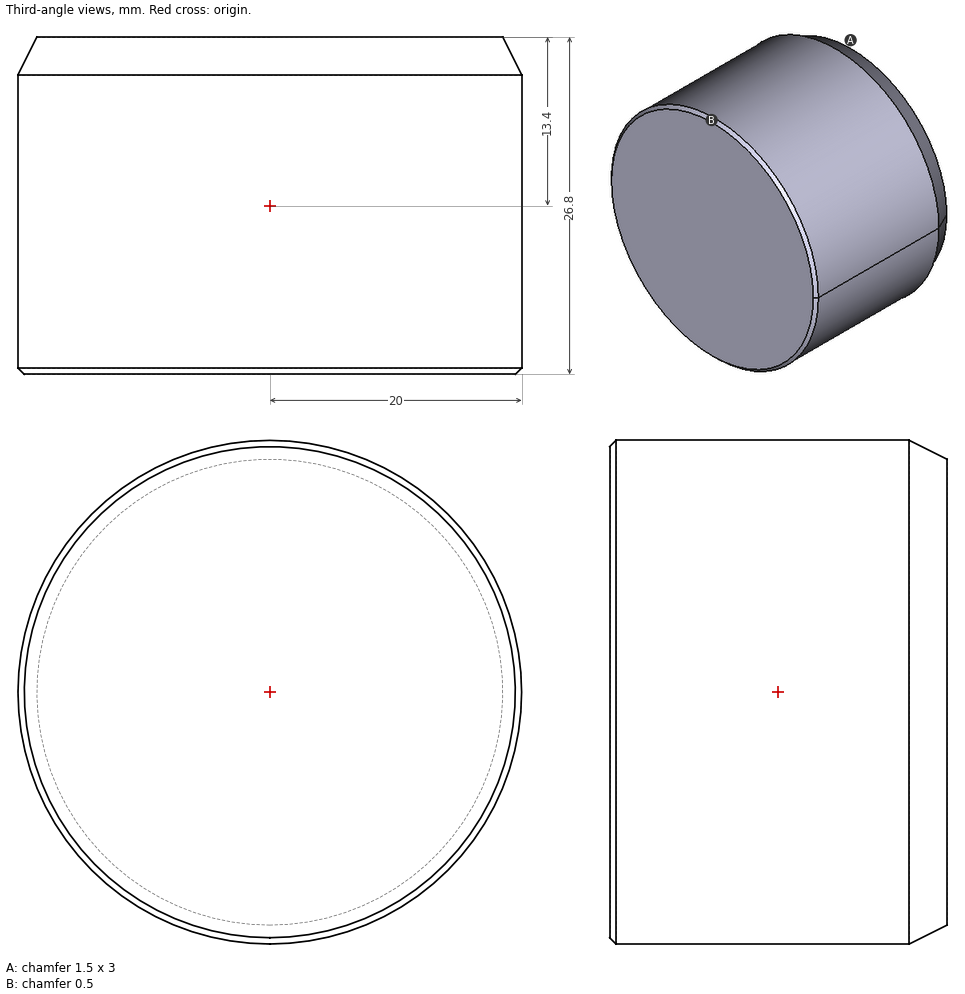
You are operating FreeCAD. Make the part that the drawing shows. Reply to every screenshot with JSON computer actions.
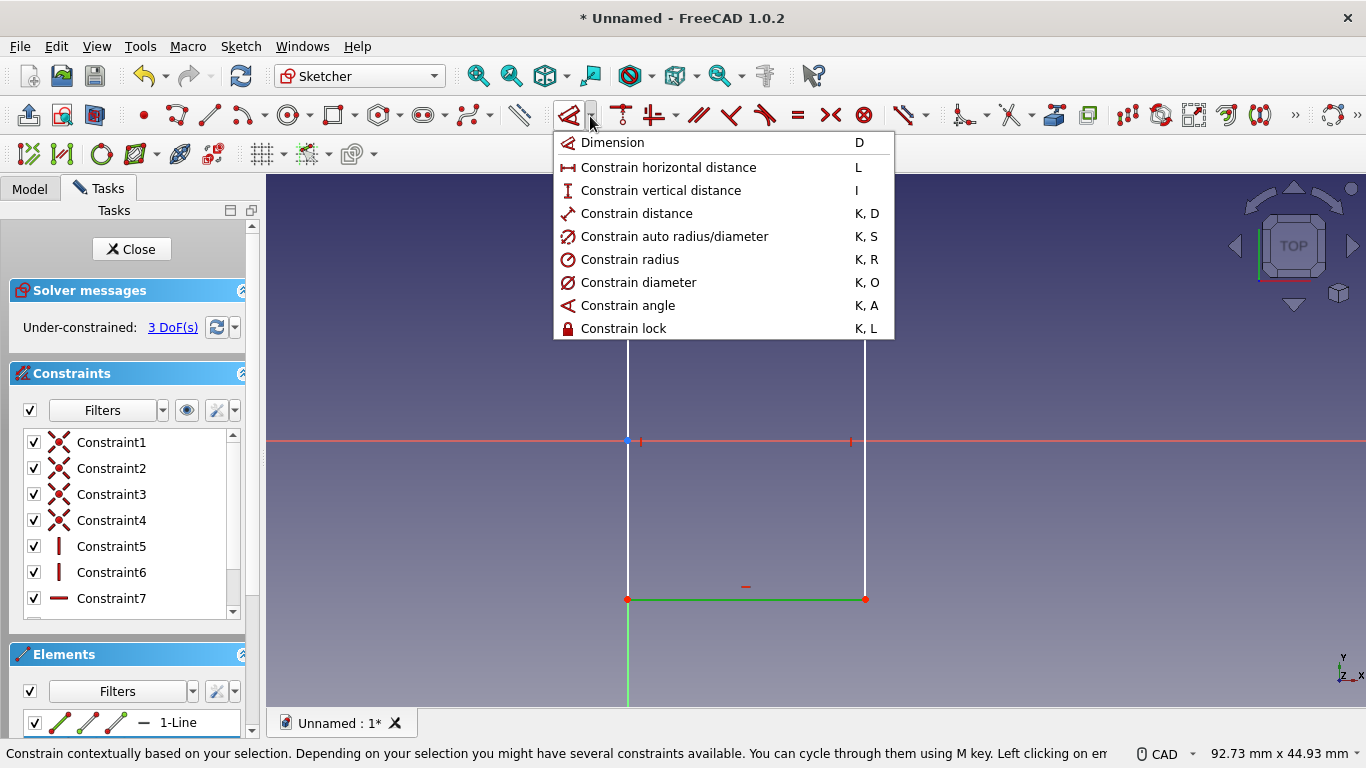
{"action": "left_click", "coordinate": [724, 168]}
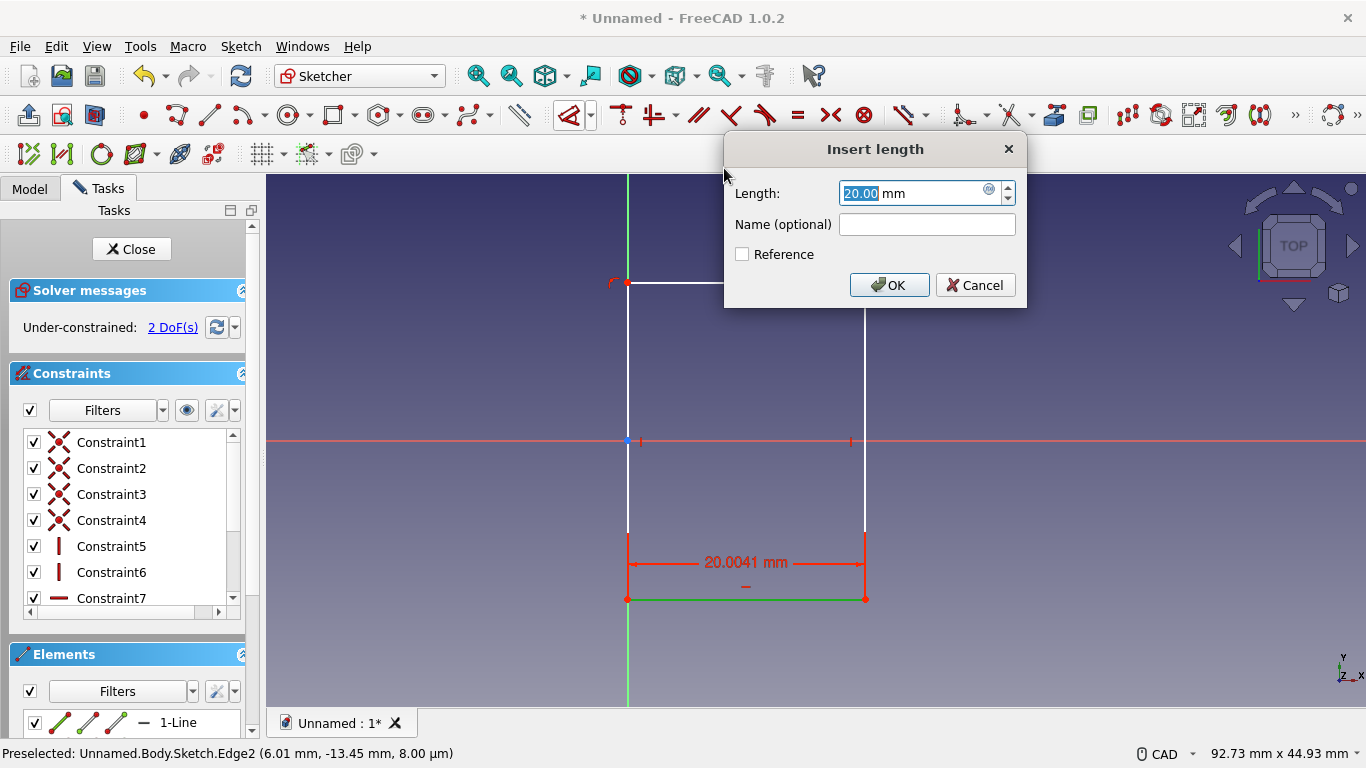
{"action": "type", "text": "20"}
{"action": "key", "text": "Return"}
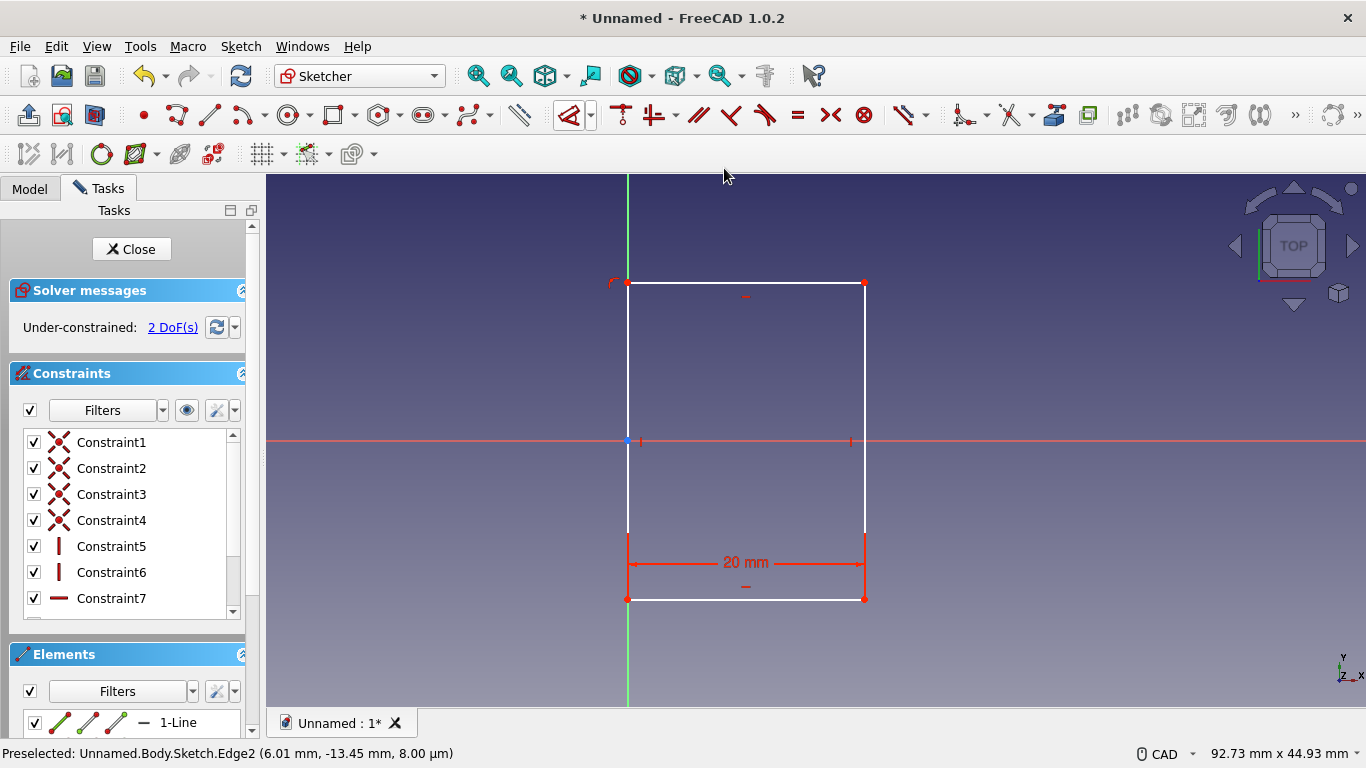
{"action": "left_click", "coordinate": [628, 378]}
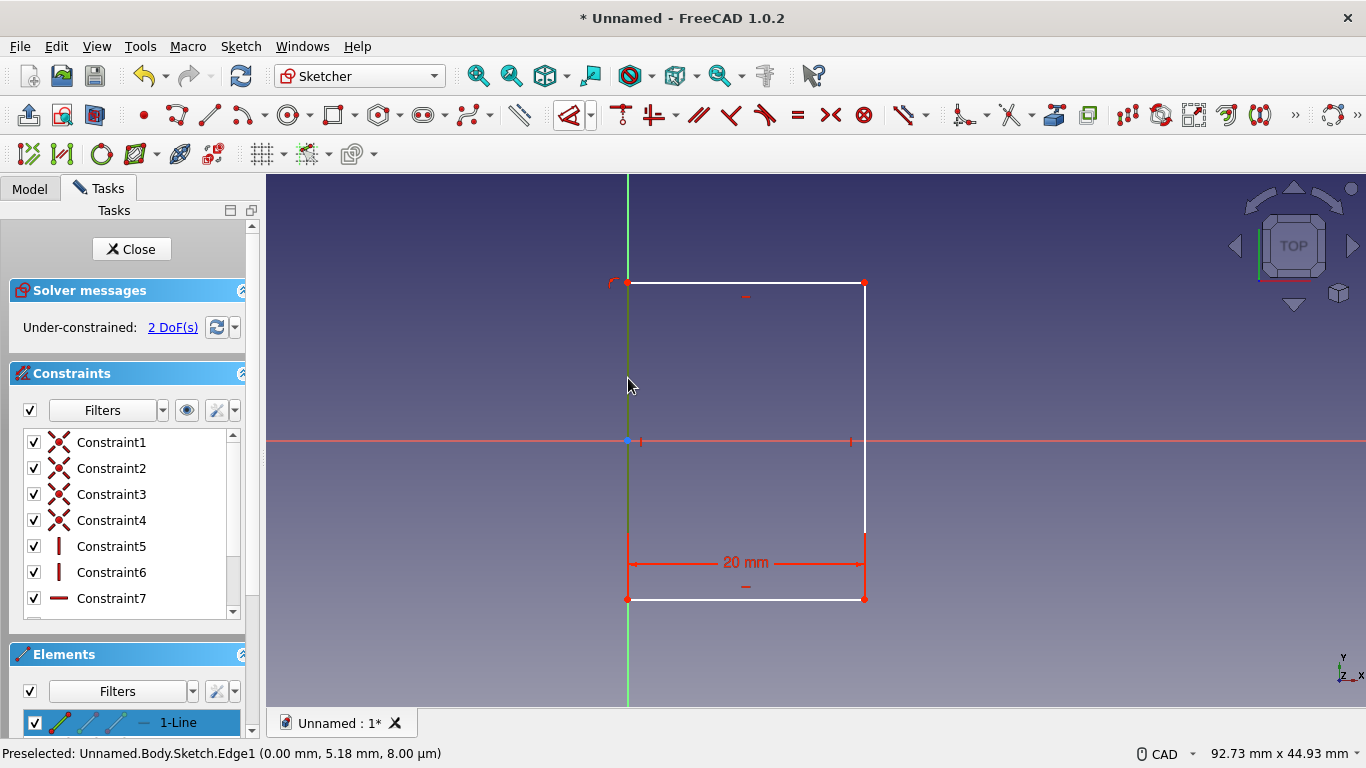
{"action": "left_click", "coordinate": [590, 116]}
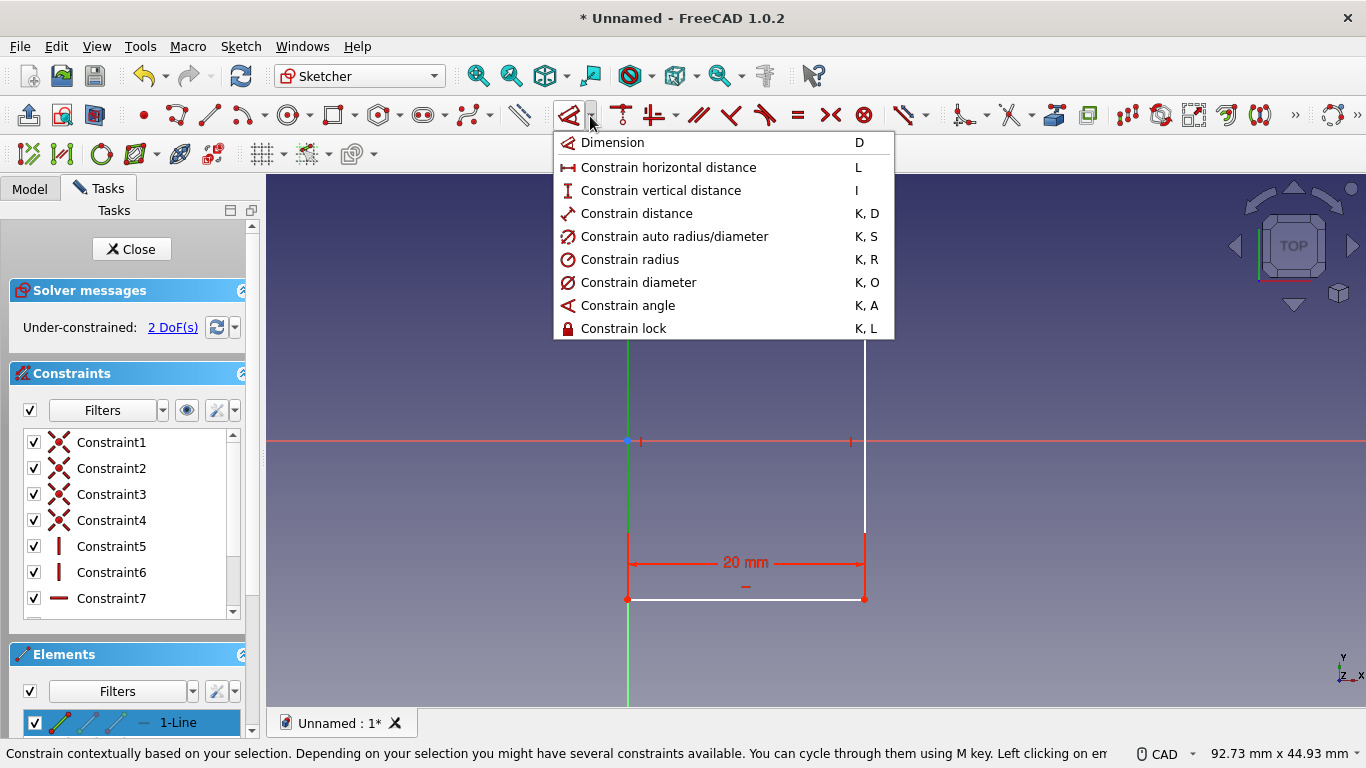
{"action": "left_click", "coordinate": [724, 190]}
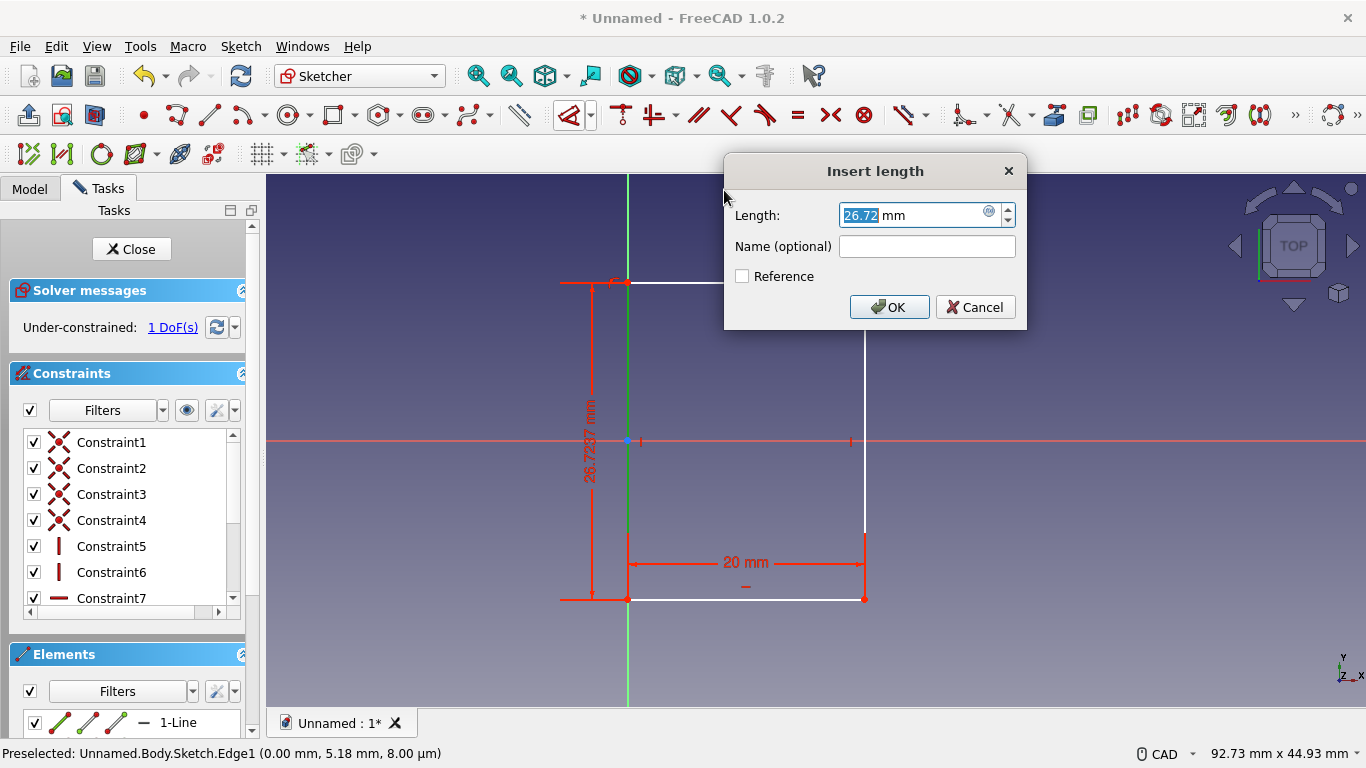
{"action": "type", "text": "26.8"}
{"action": "key", "text": "Return"}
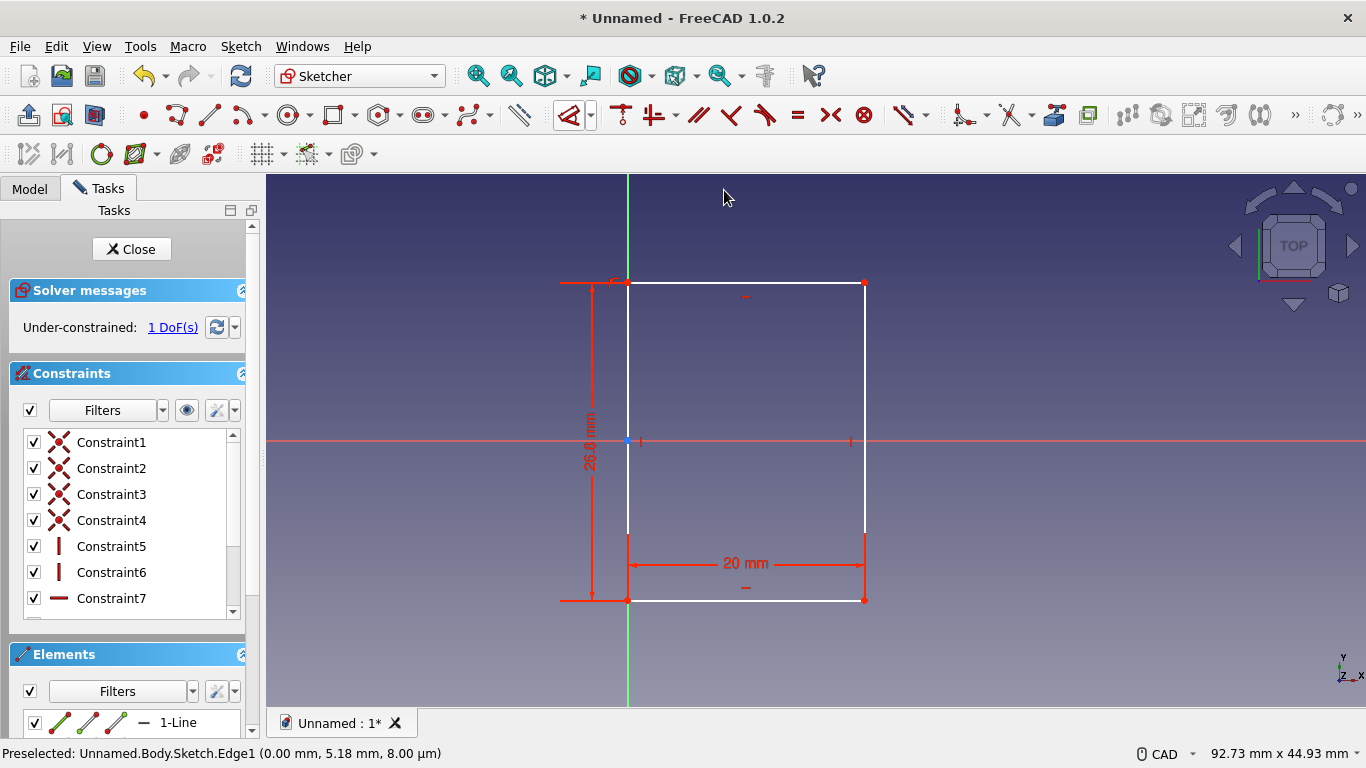
{"action": "left_click", "coordinate": [628, 283]}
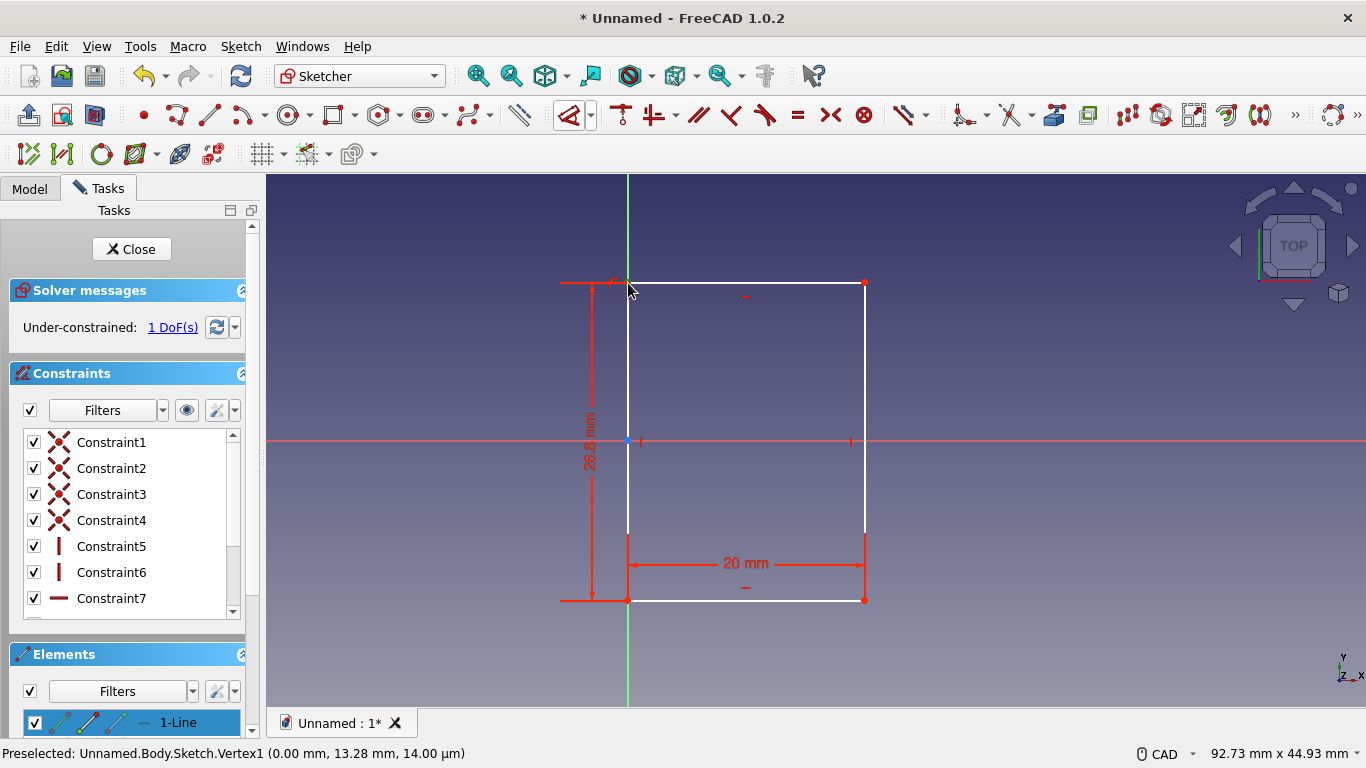
{"action": "key", "text": "i"}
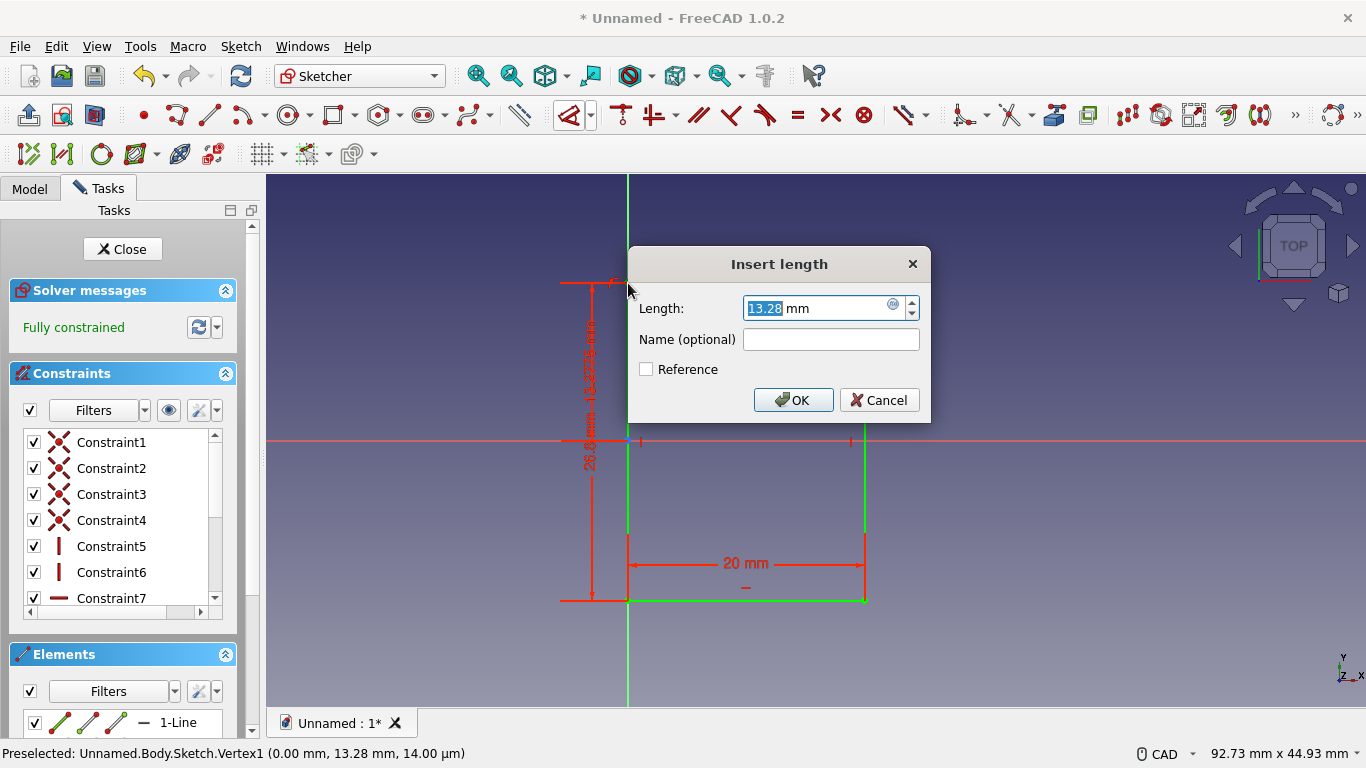
{"action": "type", "text": "13.4"}
{"action": "key", "text": "Return"}